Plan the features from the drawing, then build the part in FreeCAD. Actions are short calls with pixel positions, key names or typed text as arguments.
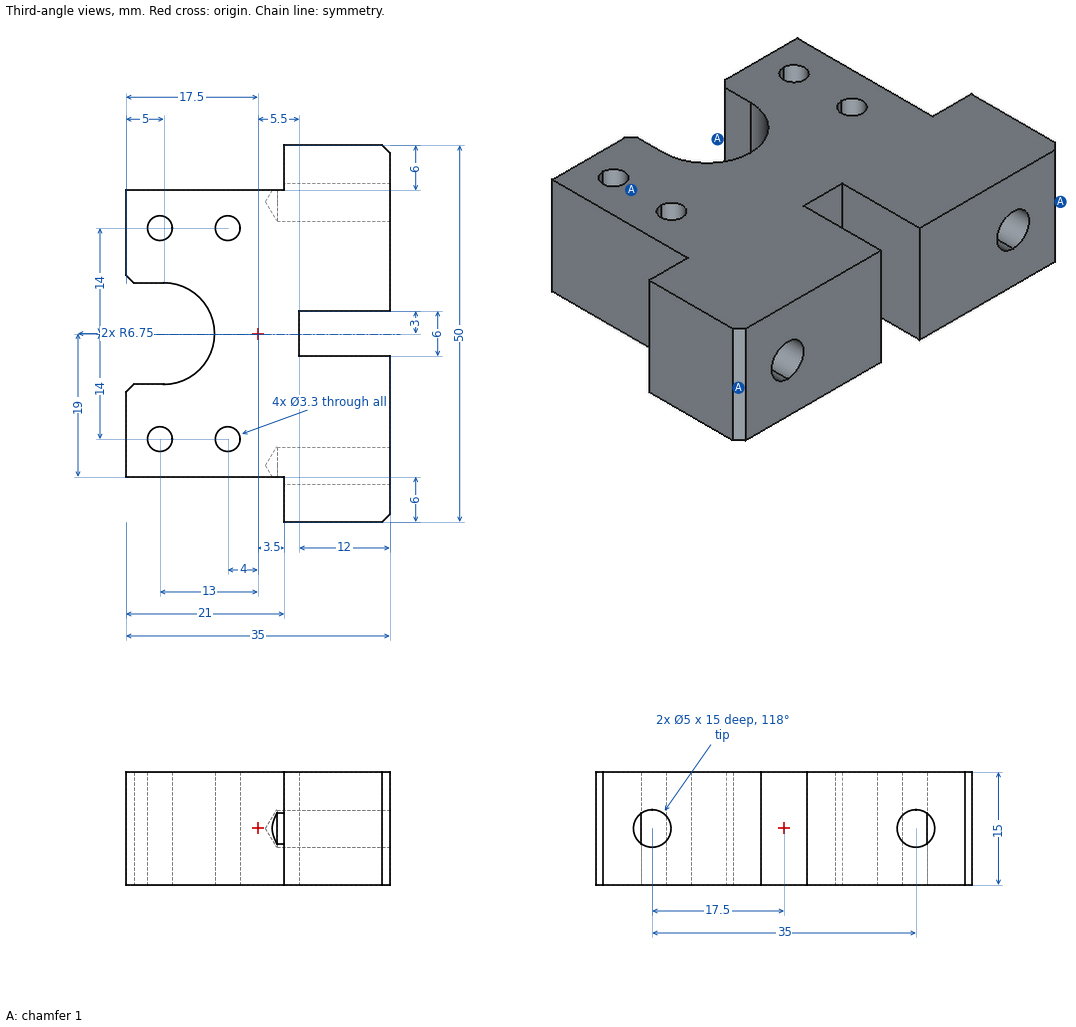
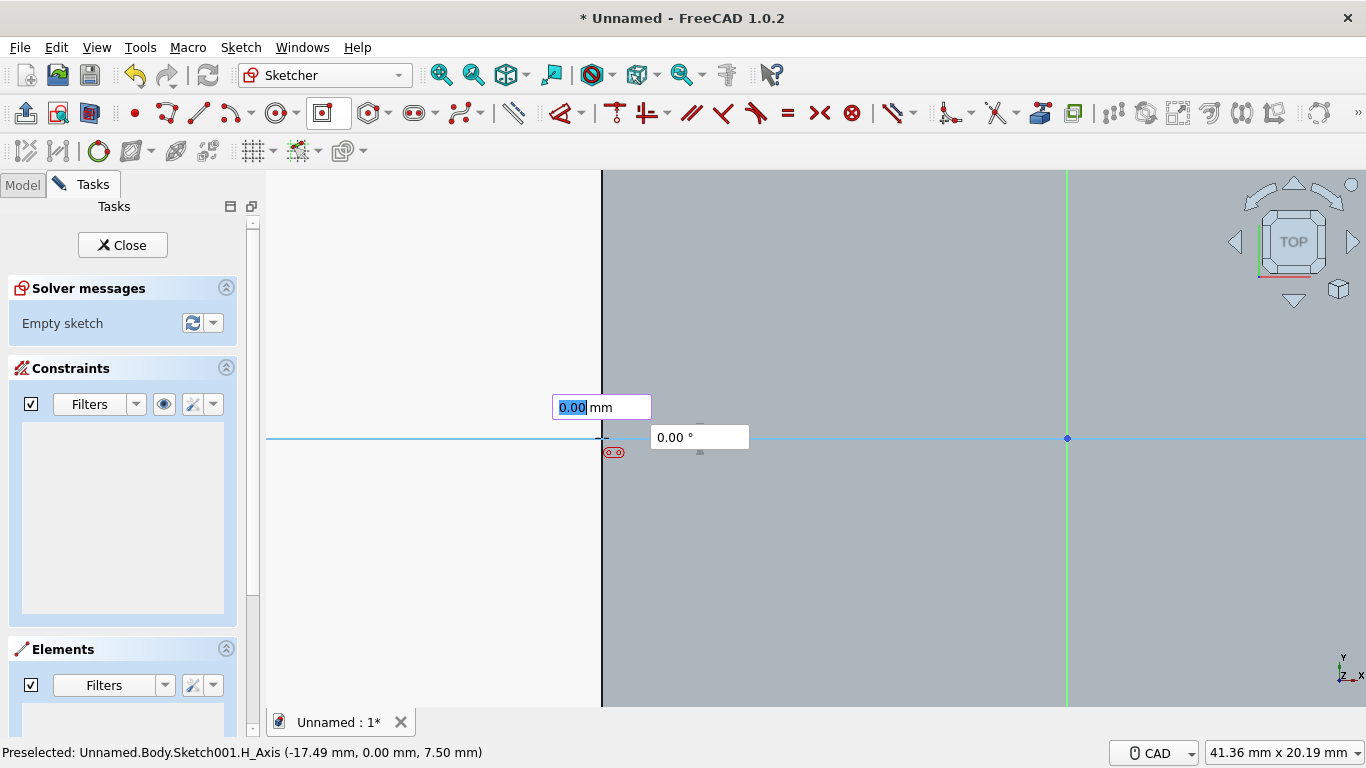
click(735, 430)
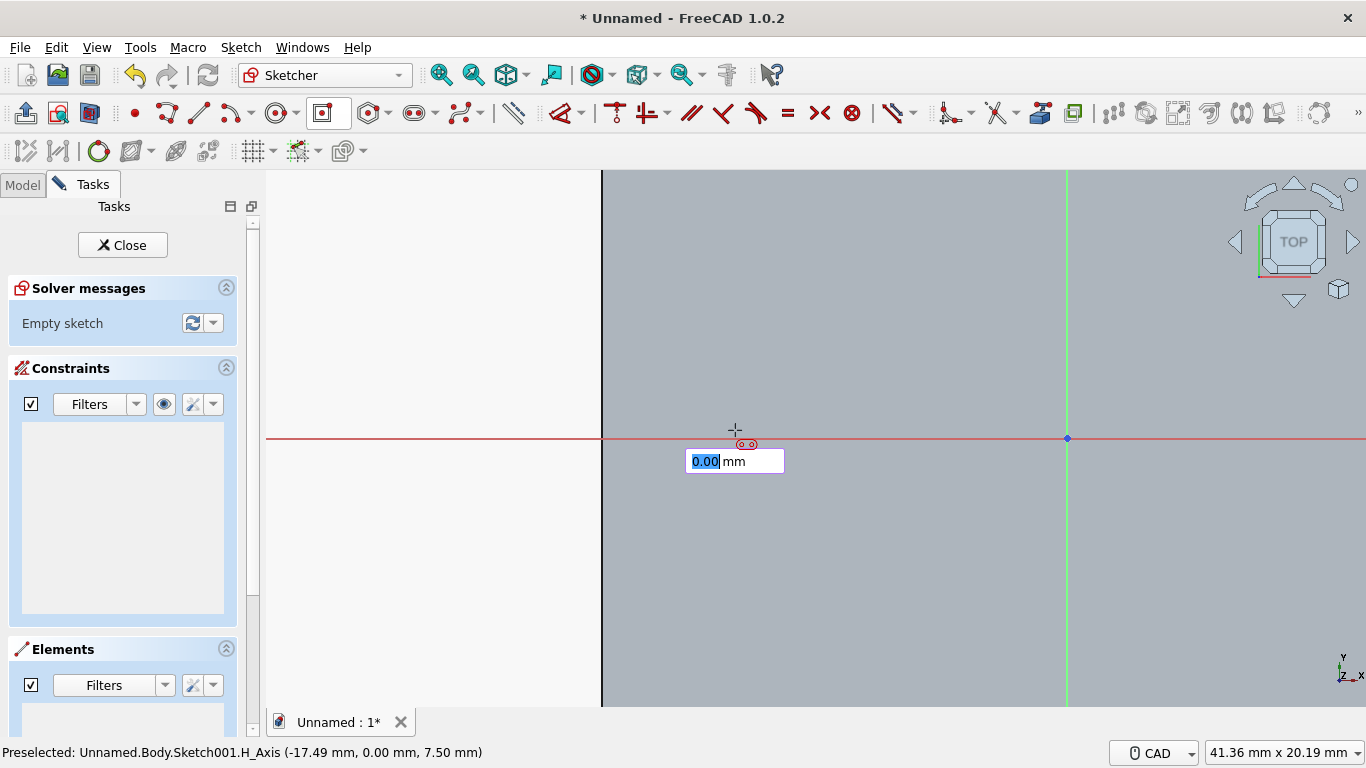
click(668, 259)
key(Escape)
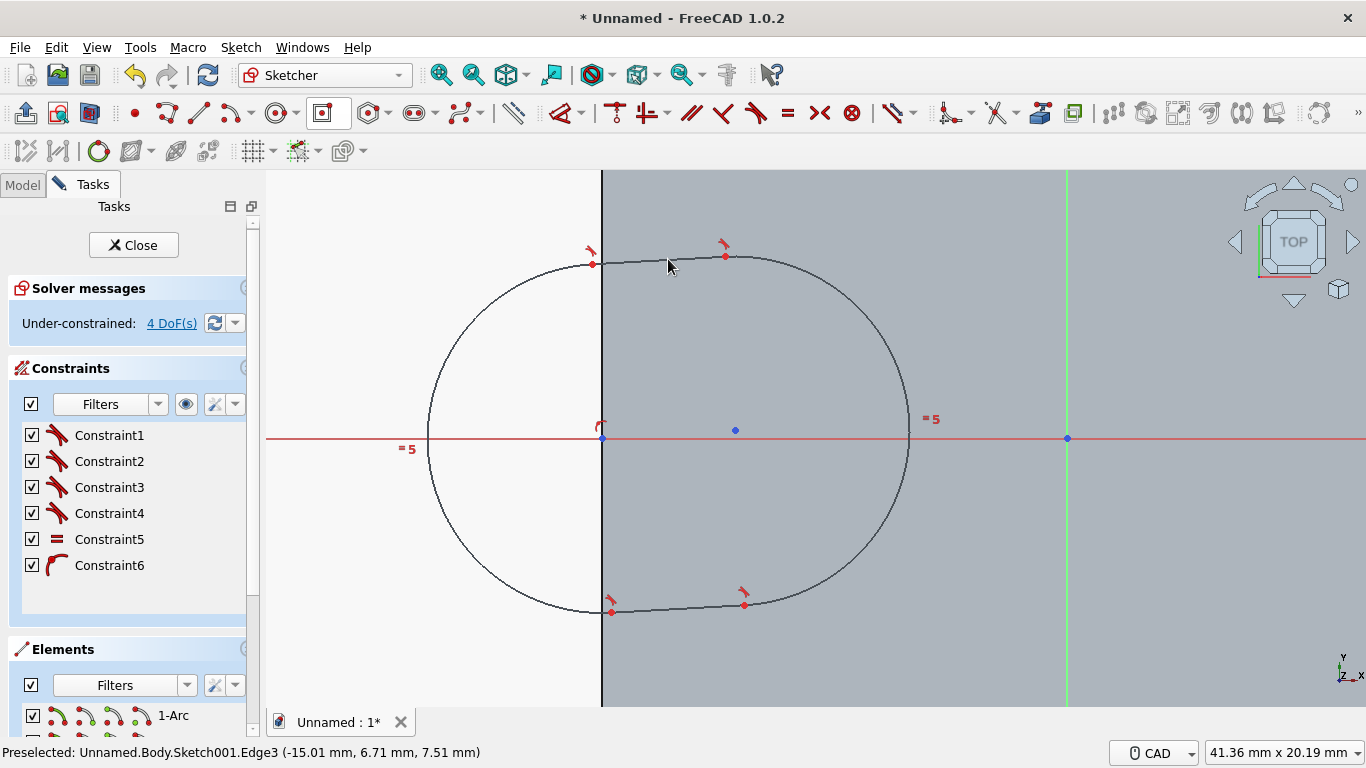
click(632, 262)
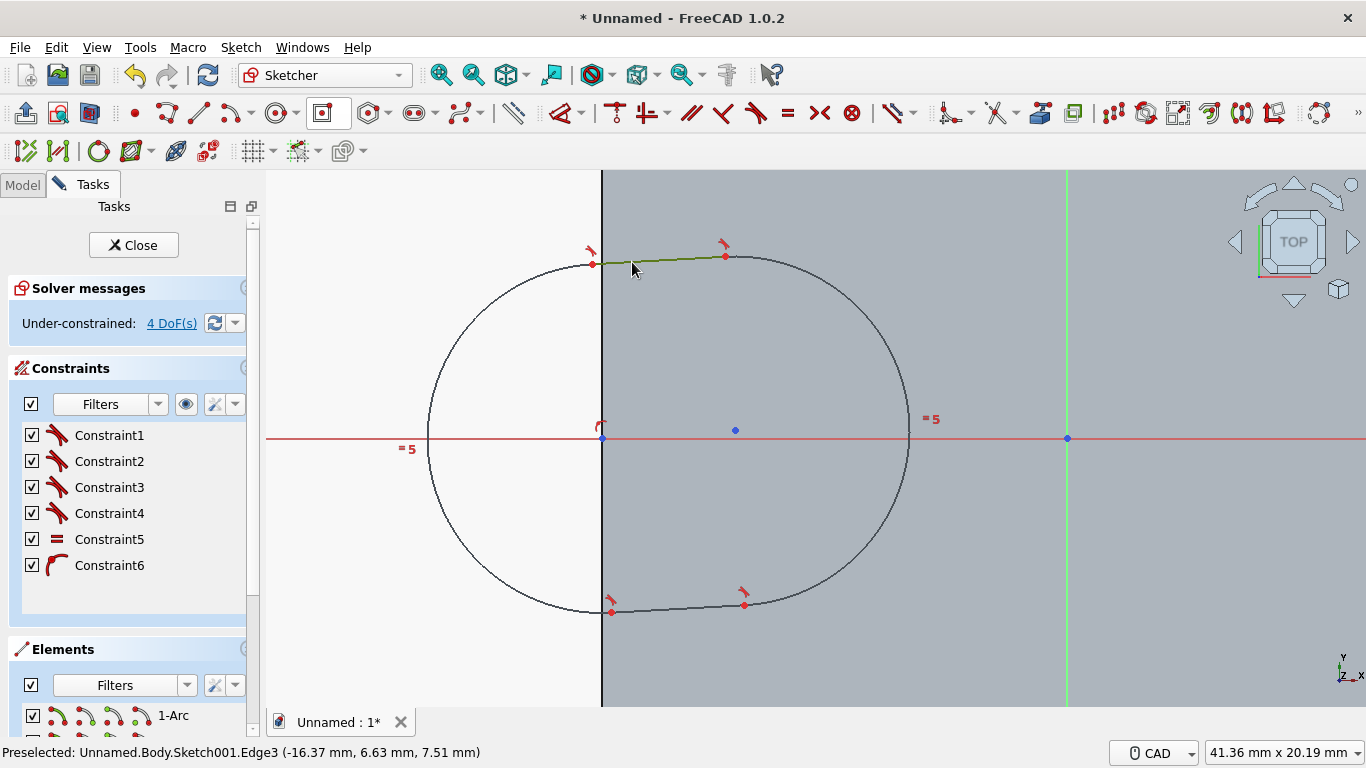
click(670, 114)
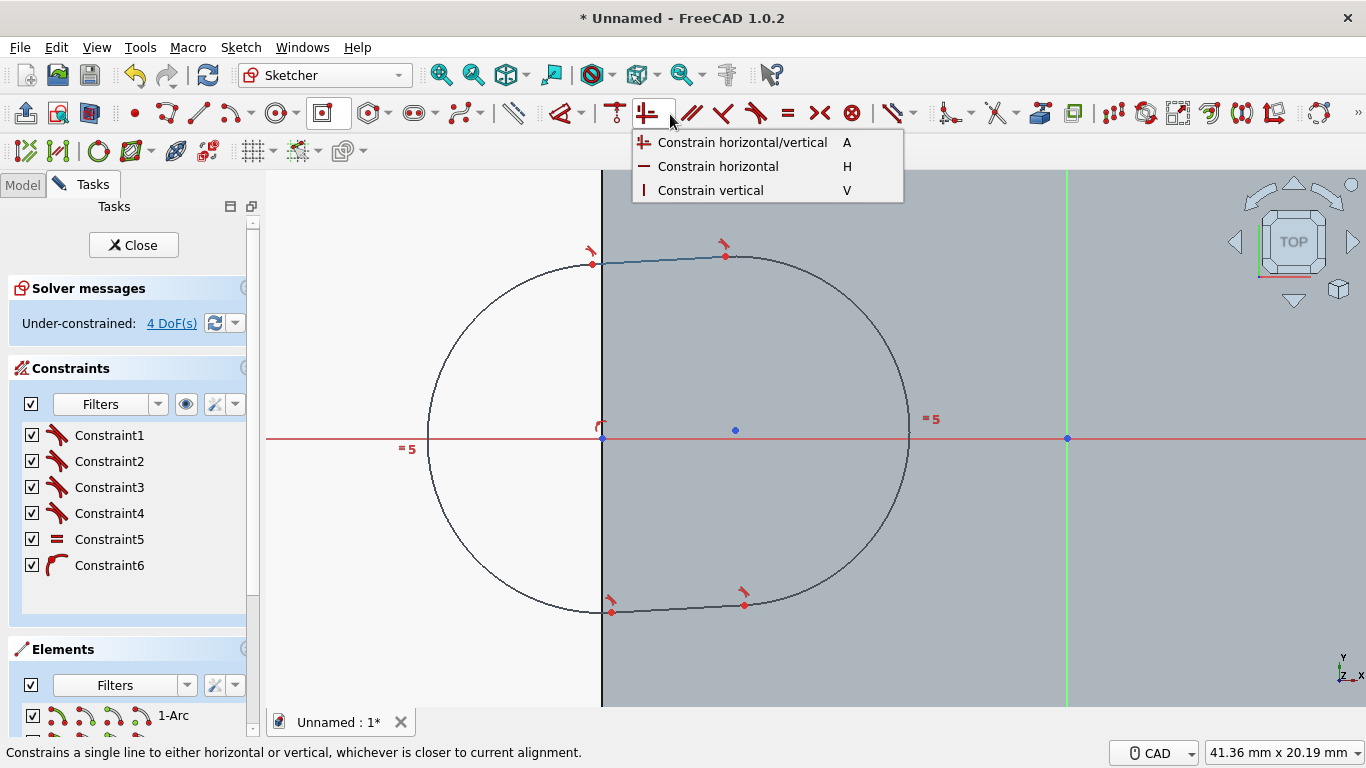
click(768, 166)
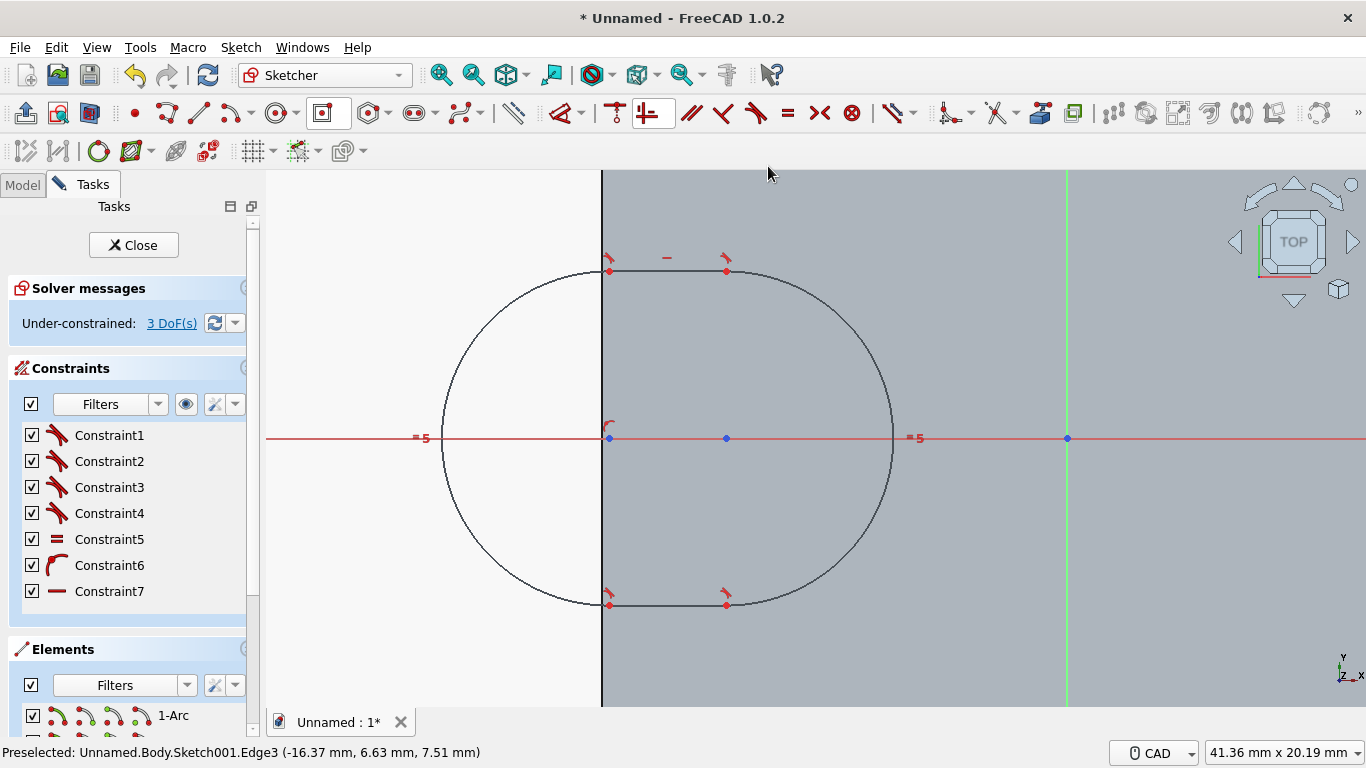
click(560, 114)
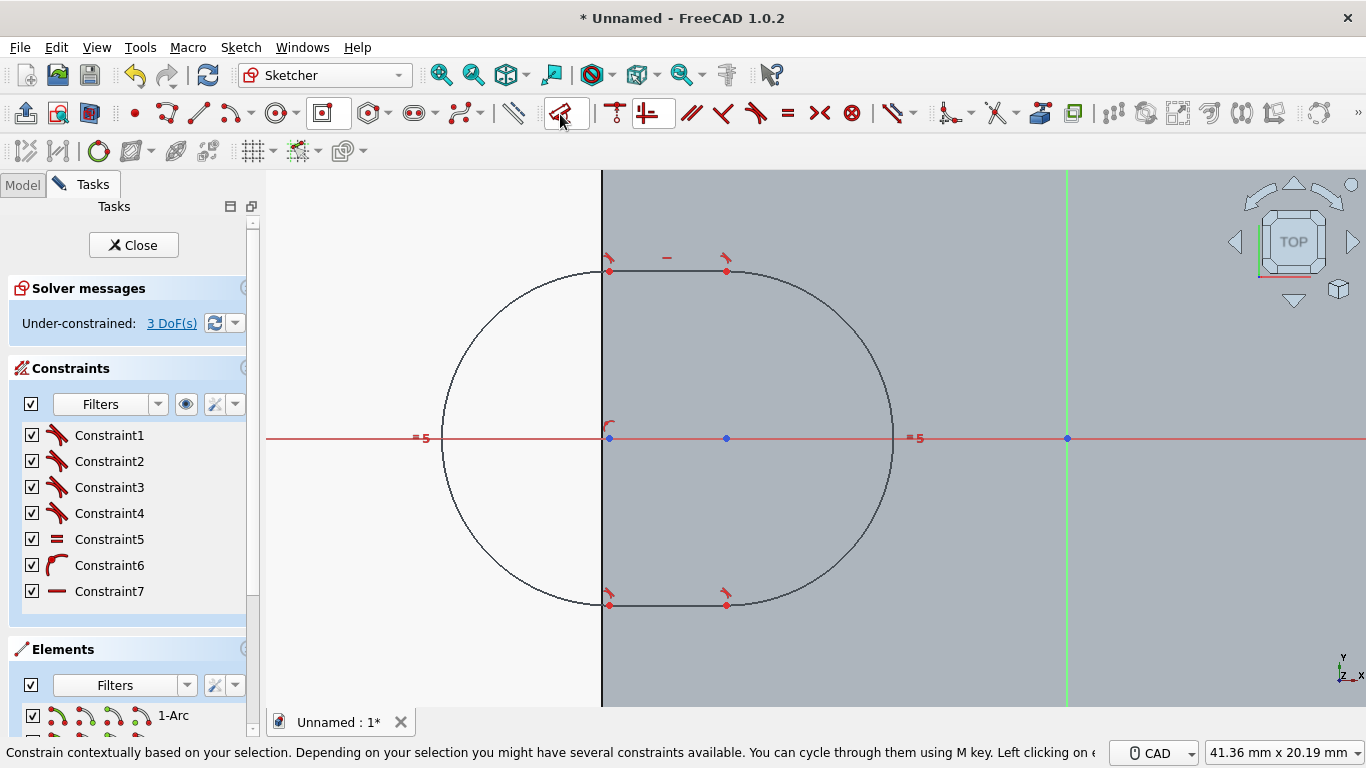
click(474, 340)
click(448, 321)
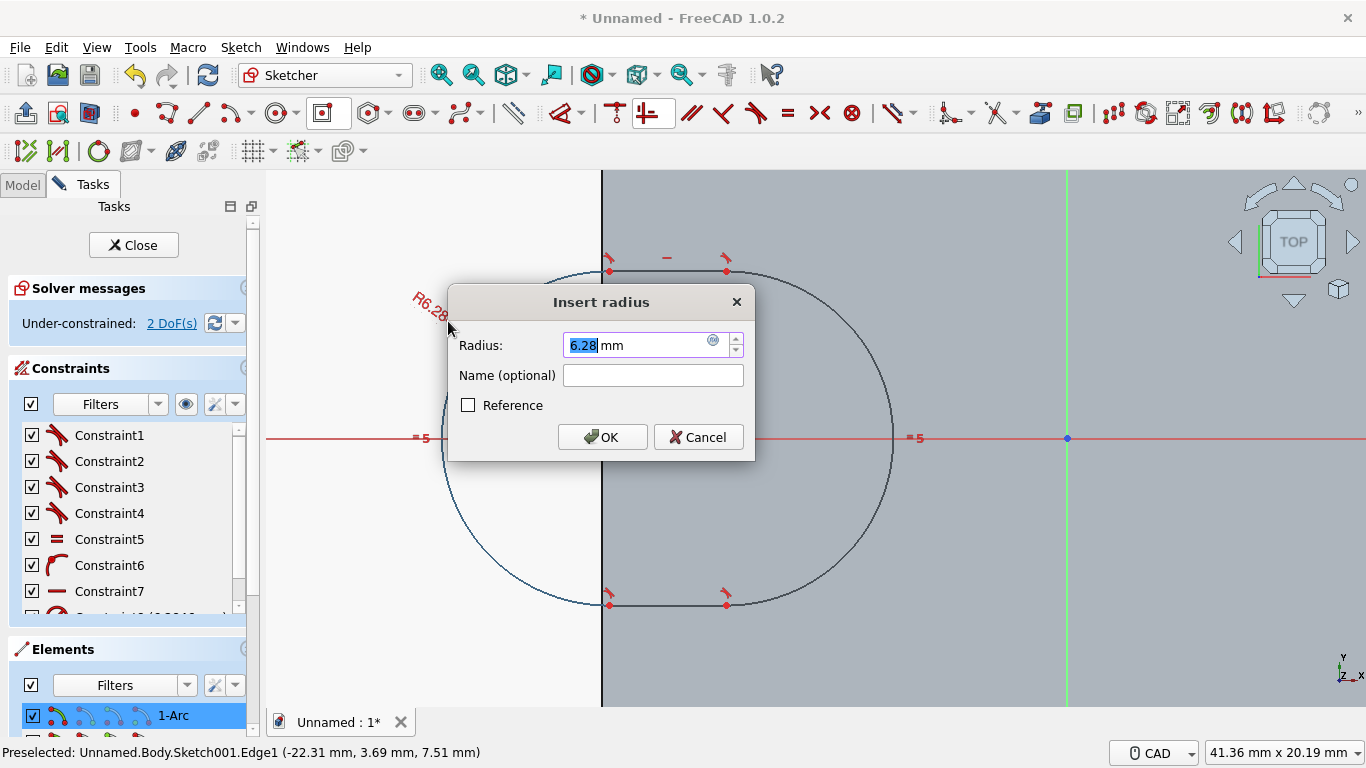
text(6.75)
key(Return)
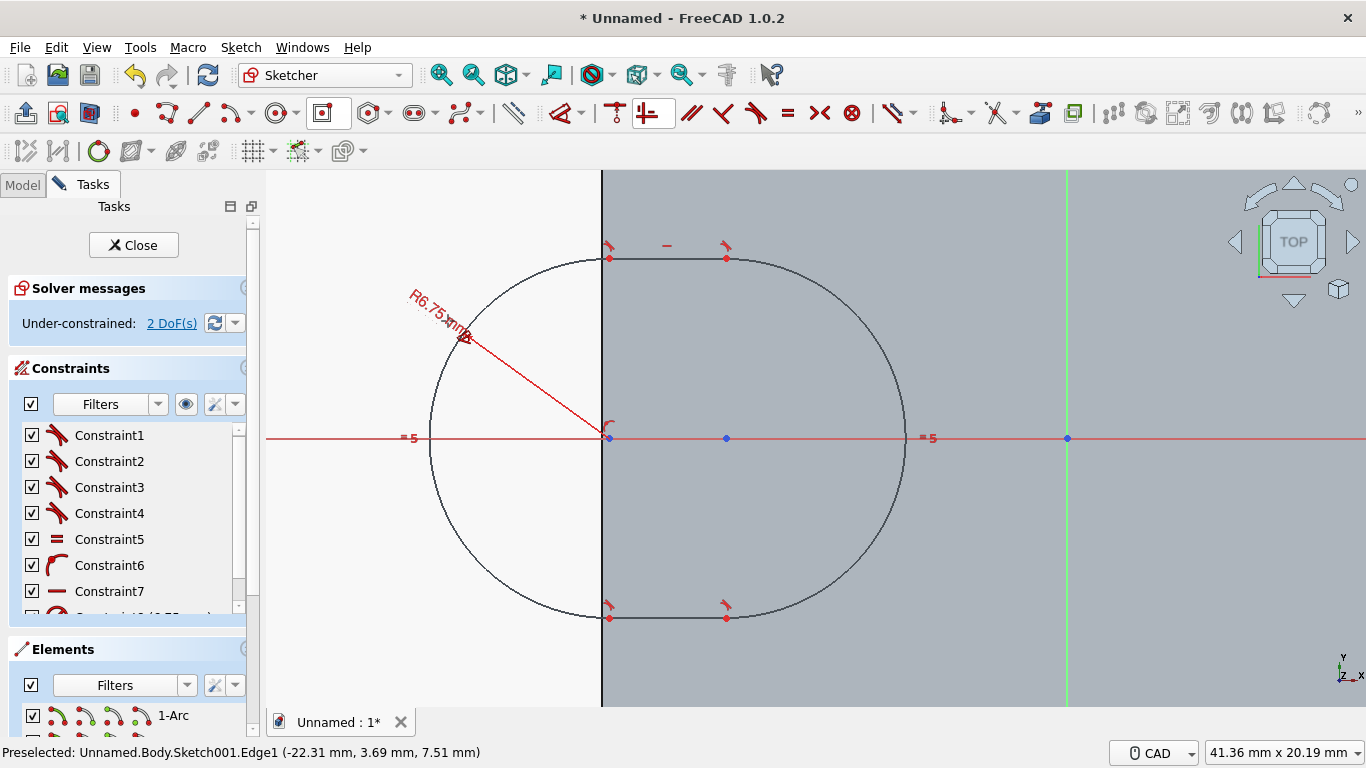
click(644, 259)
click(668, 225)